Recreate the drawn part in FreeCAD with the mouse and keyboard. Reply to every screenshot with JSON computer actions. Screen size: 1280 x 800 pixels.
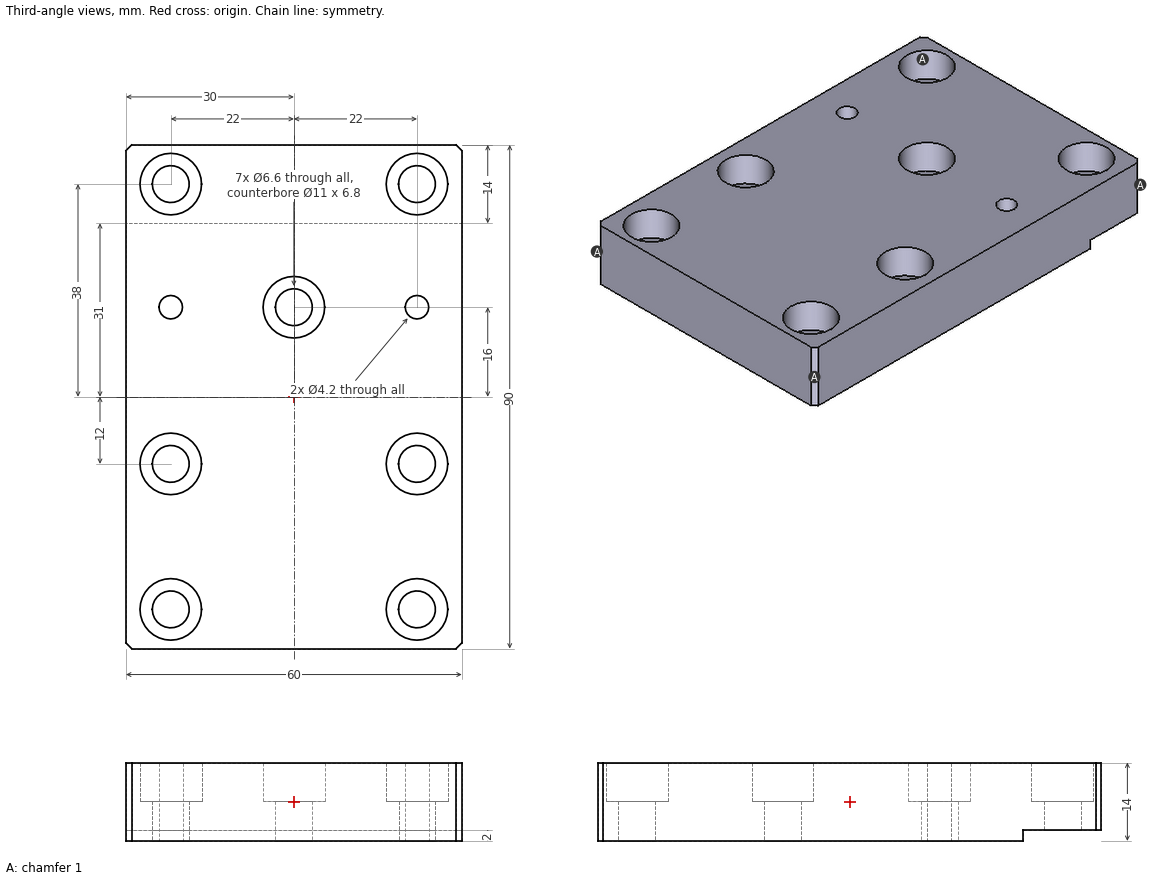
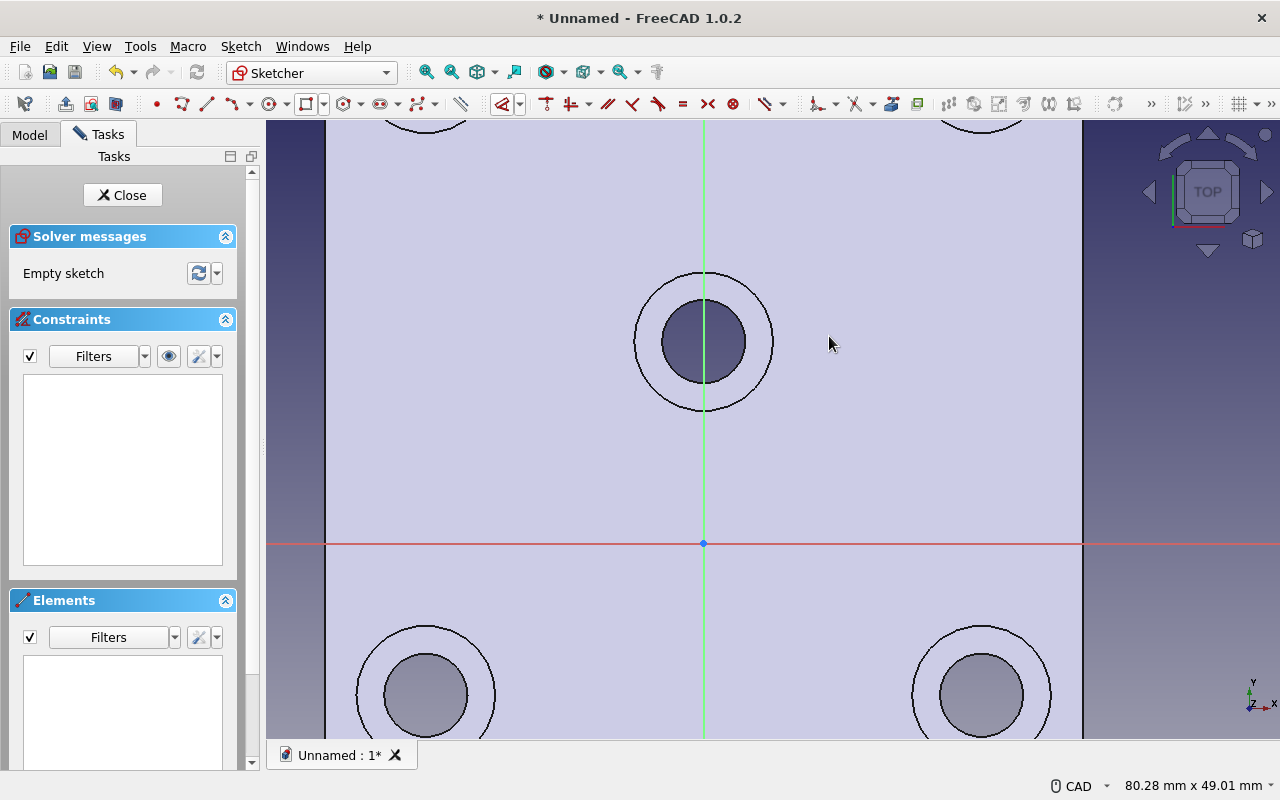
{"action": "left_click", "coordinate": [268, 104]}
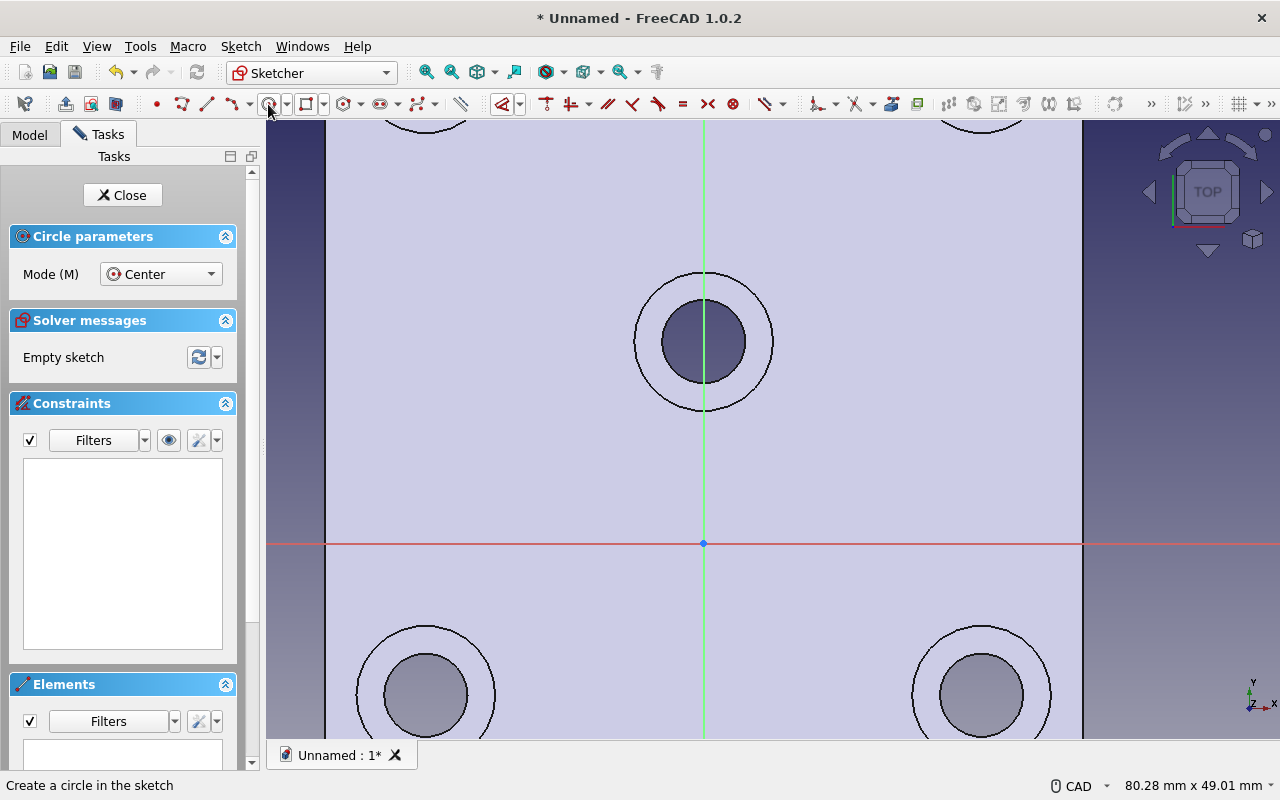
{"action": "left_click", "coordinate": [982, 342]}
{"action": "mouse_move", "coordinate": [1000, 323]}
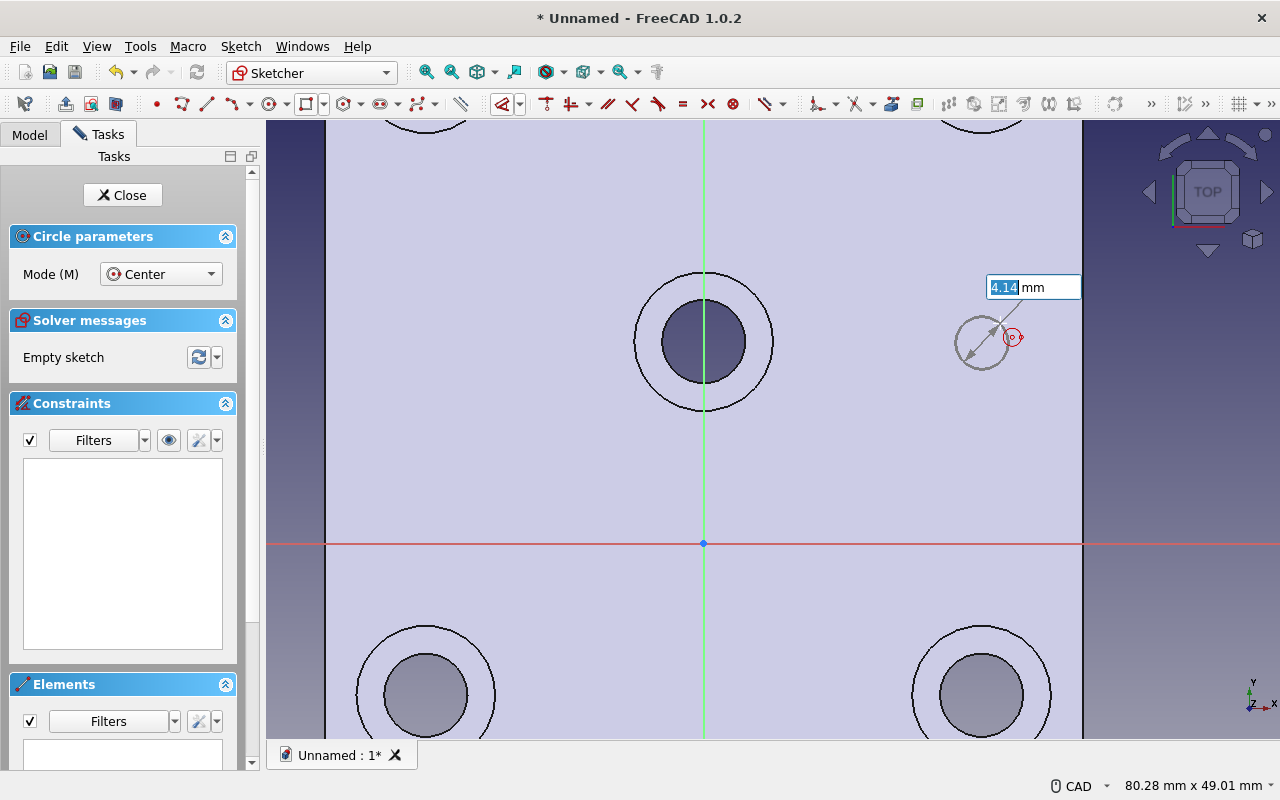
{"action": "type", "text": "4.2"}
{"action": "key", "text": "Return"}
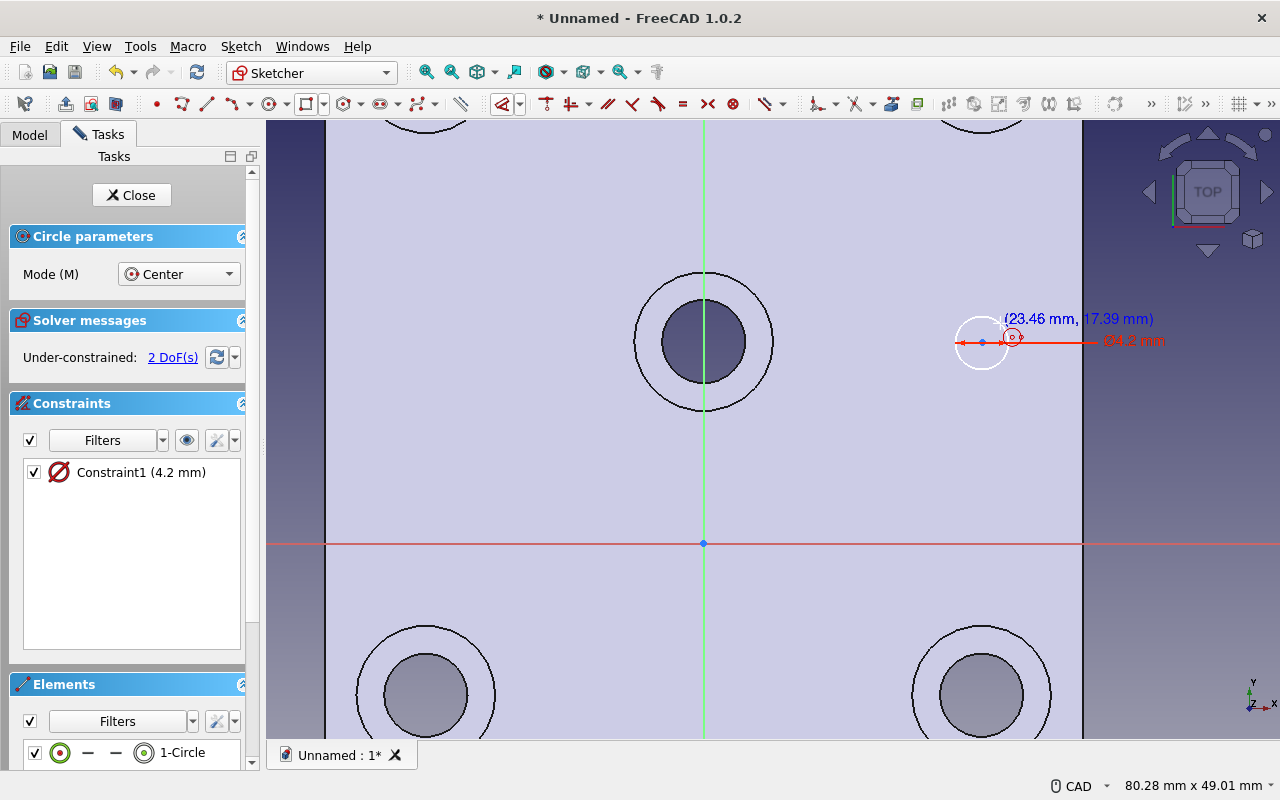
{"action": "left_click", "coordinate": [426, 342]}
{"action": "mouse_move", "coordinate": [445, 323]}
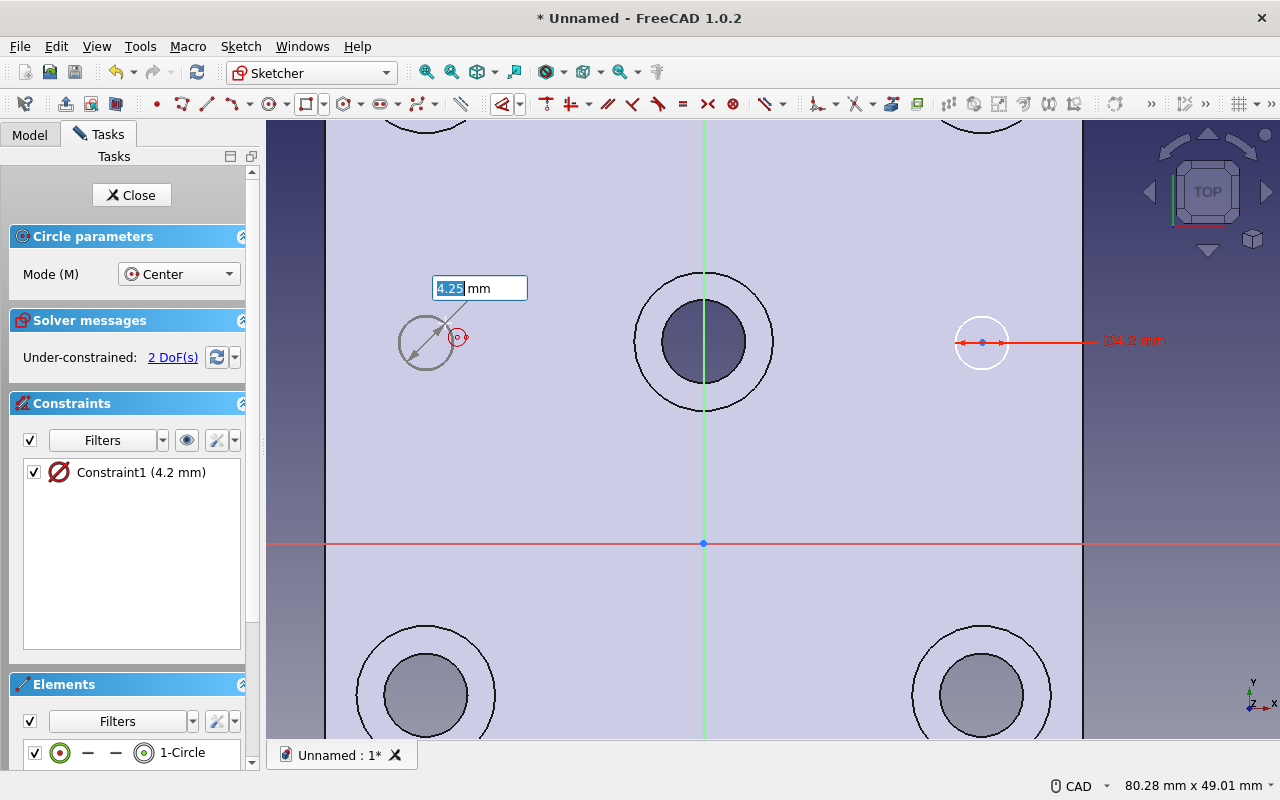
{"action": "type", "text": "4.2"}
{"action": "key", "text": "Return"}
{"action": "key", "text": "Escape"}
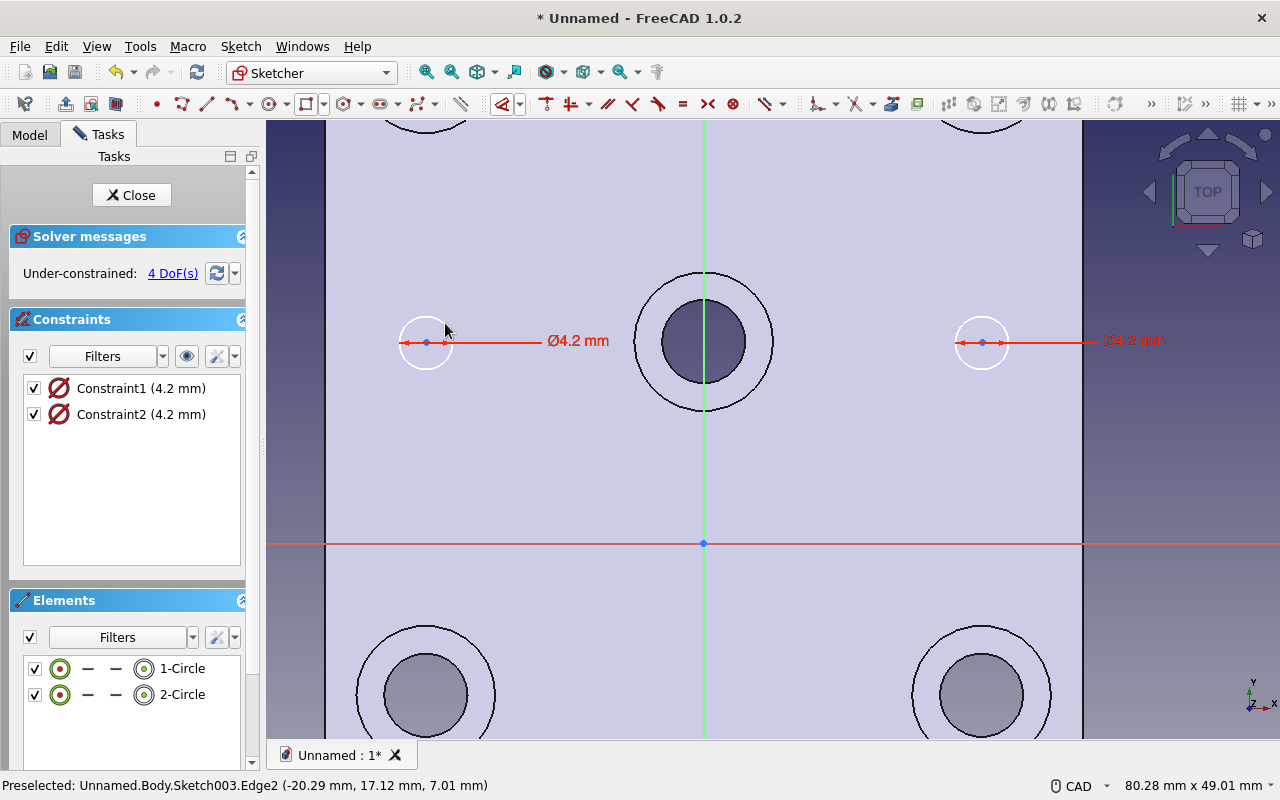
{"action": "left_click", "coordinate": [982, 343]}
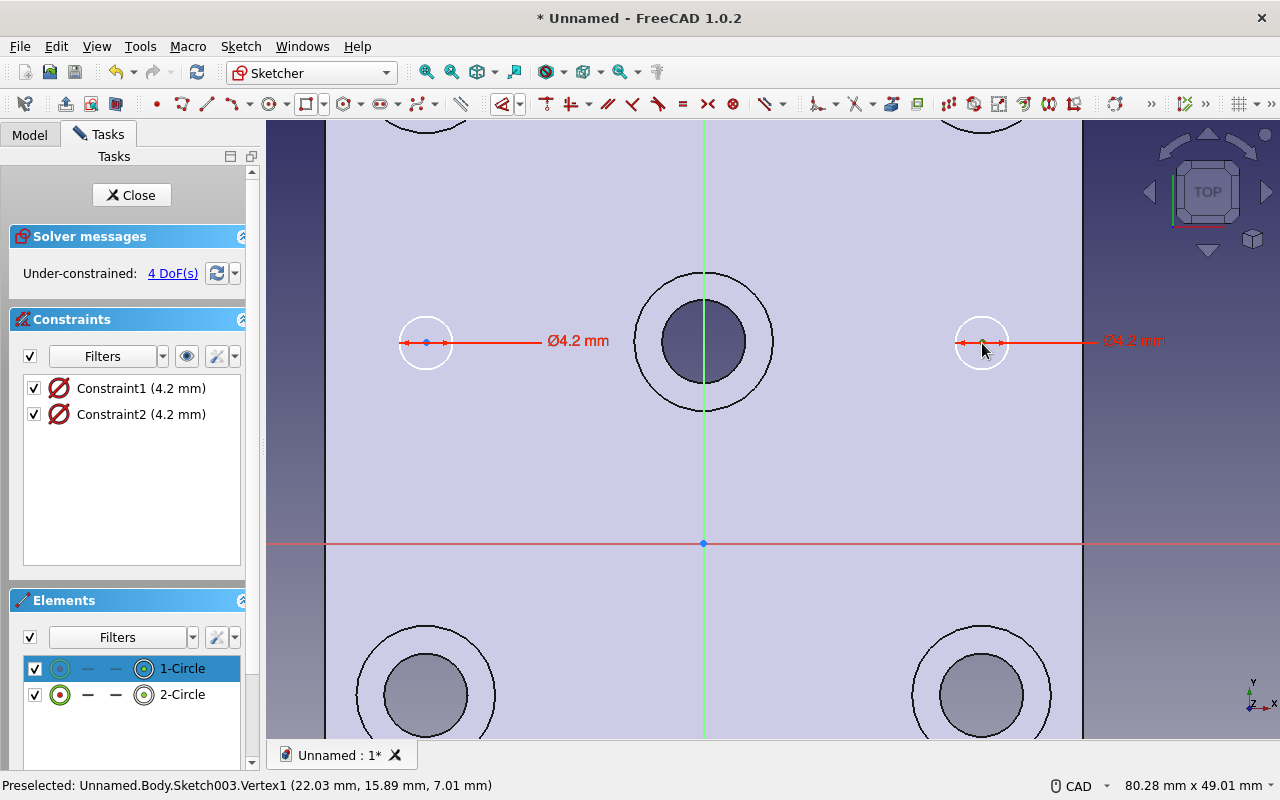
{"action": "left_click", "coordinate": [426, 343]}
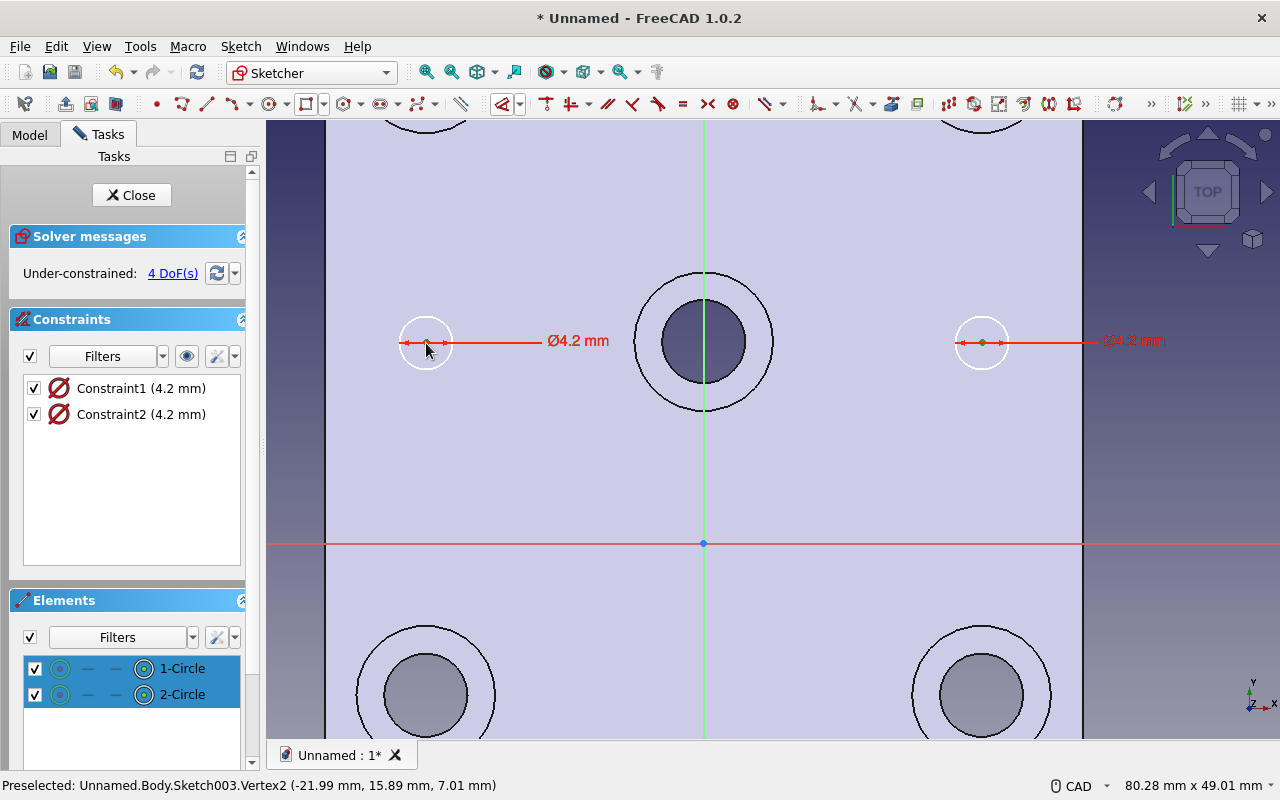
{"action": "left_click", "coordinate": [704, 671]}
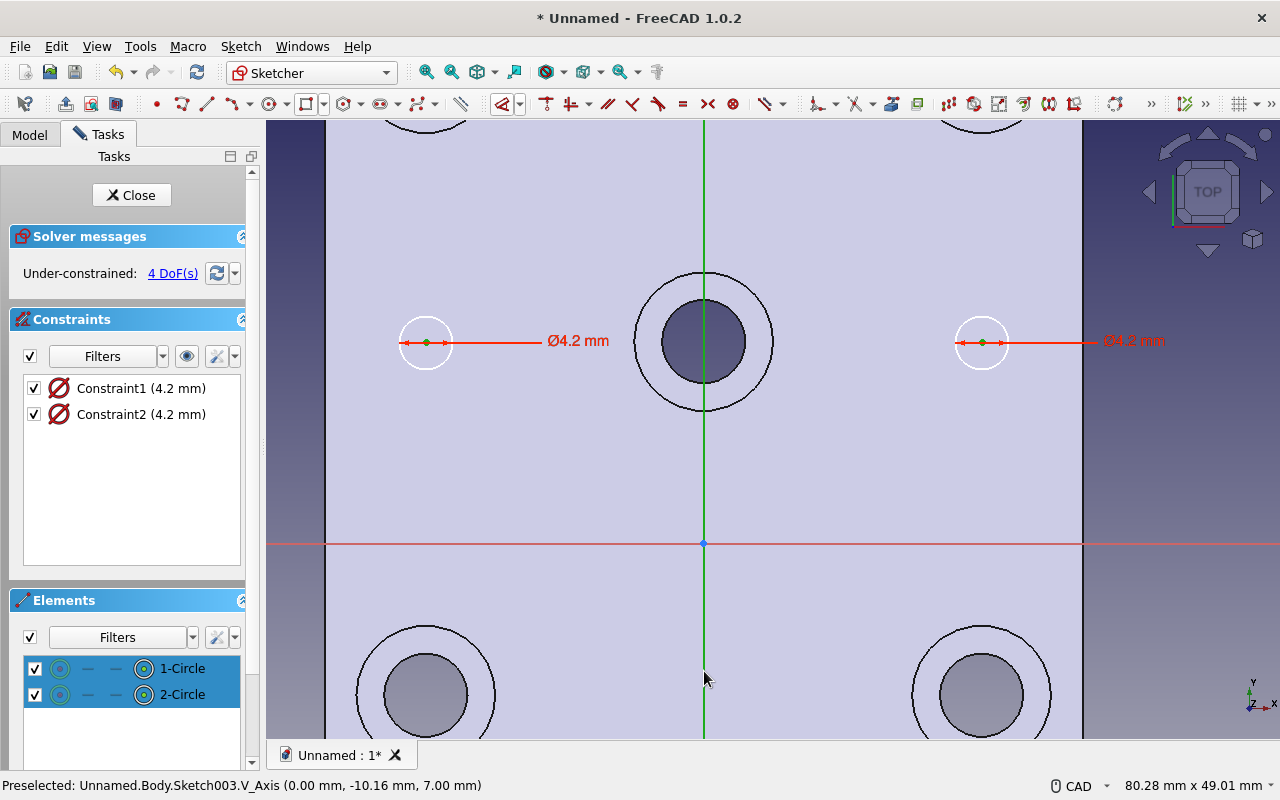
{"action": "left_click", "coordinate": [708, 104]}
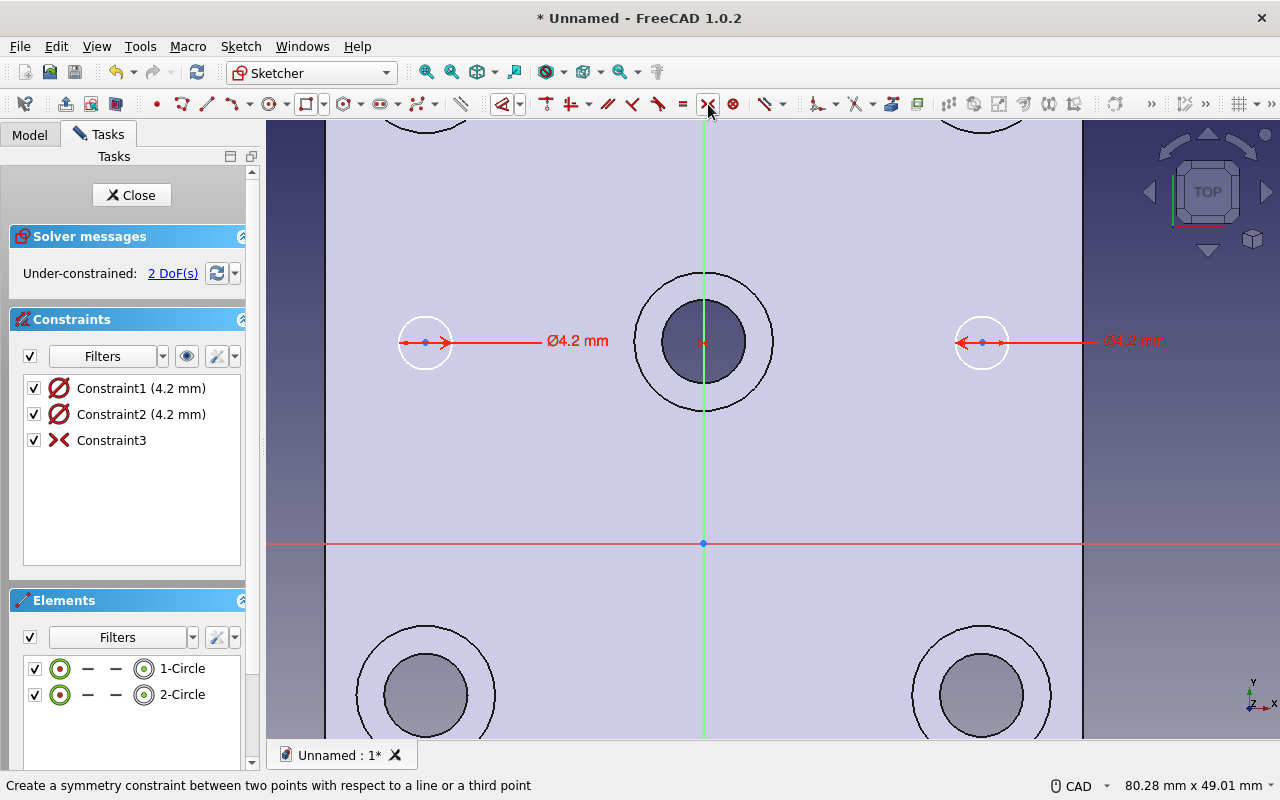
{"action": "left_click", "coordinate": [982, 343]}